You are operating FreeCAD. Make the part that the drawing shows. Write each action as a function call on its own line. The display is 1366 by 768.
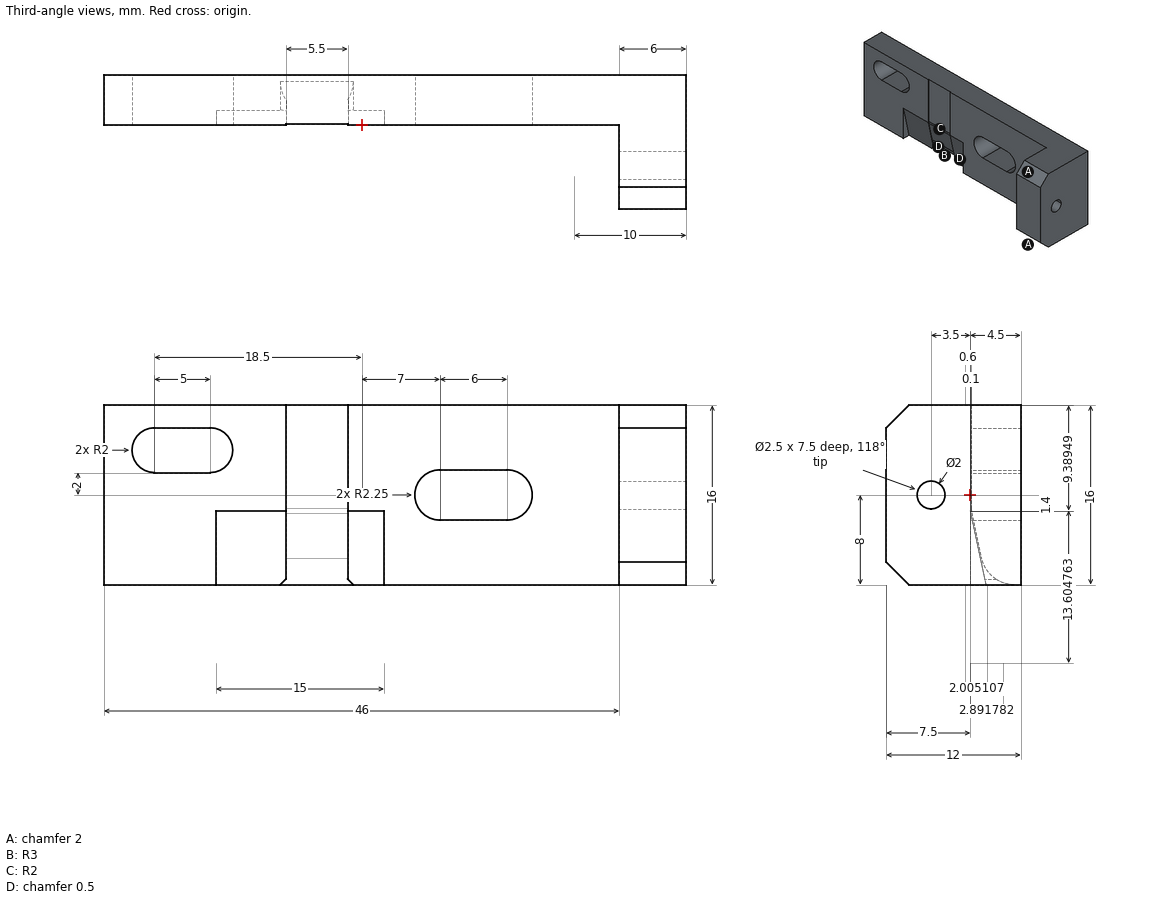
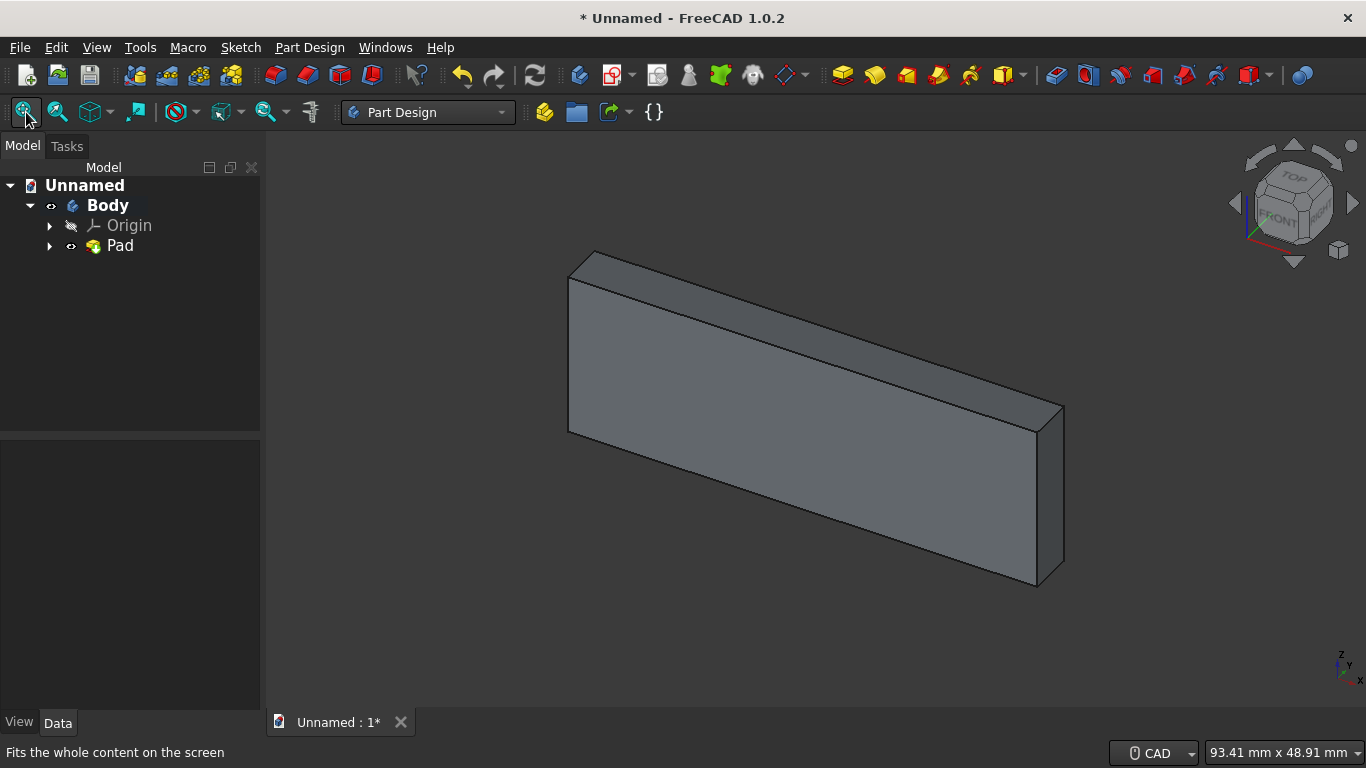
click(1051, 474)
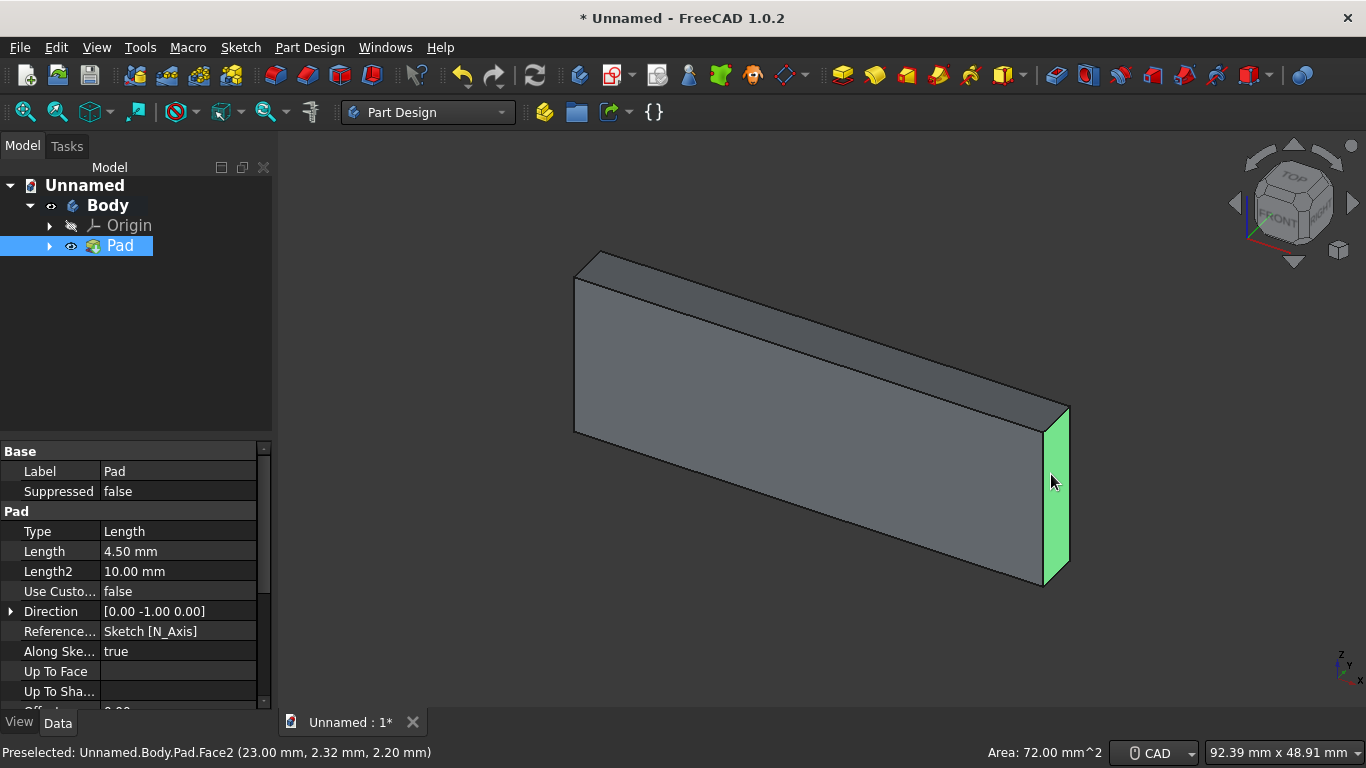
click(612, 76)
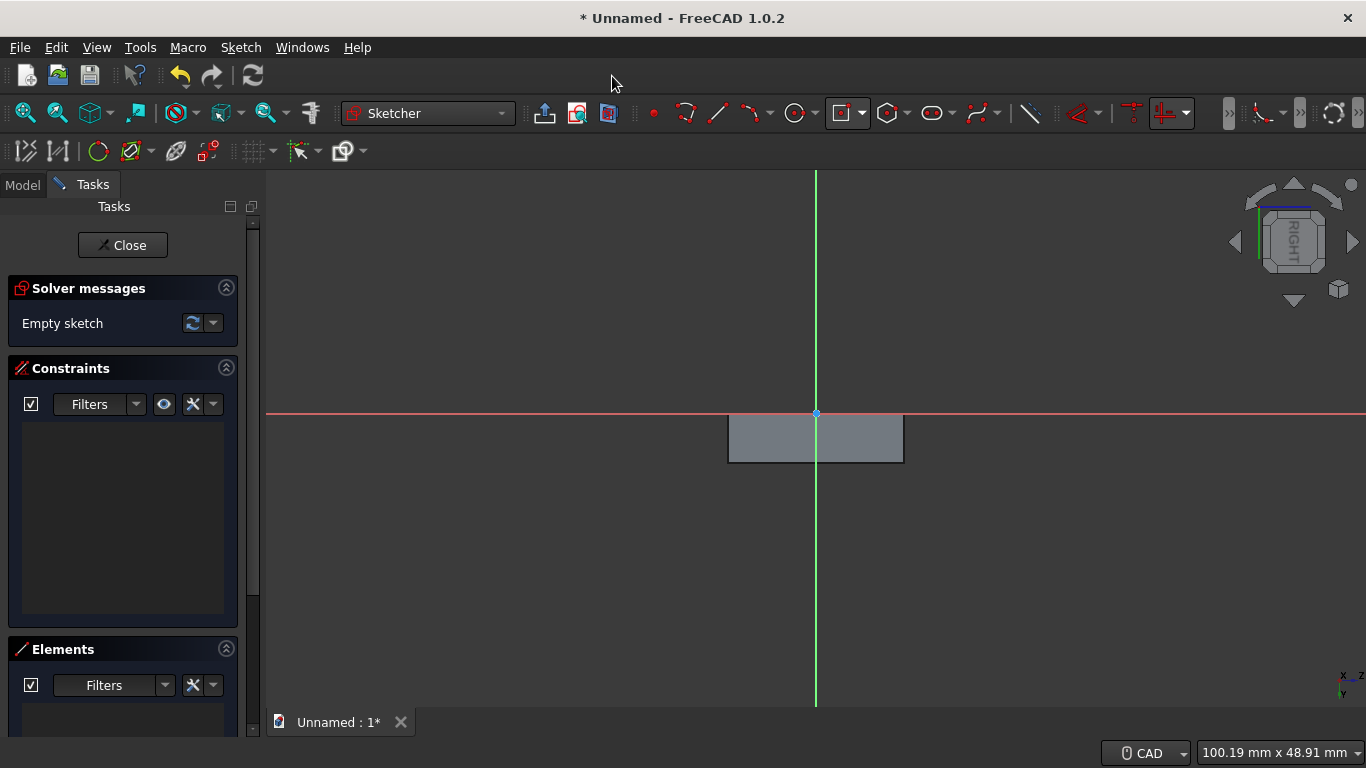
scroll(856, 373, up, 5)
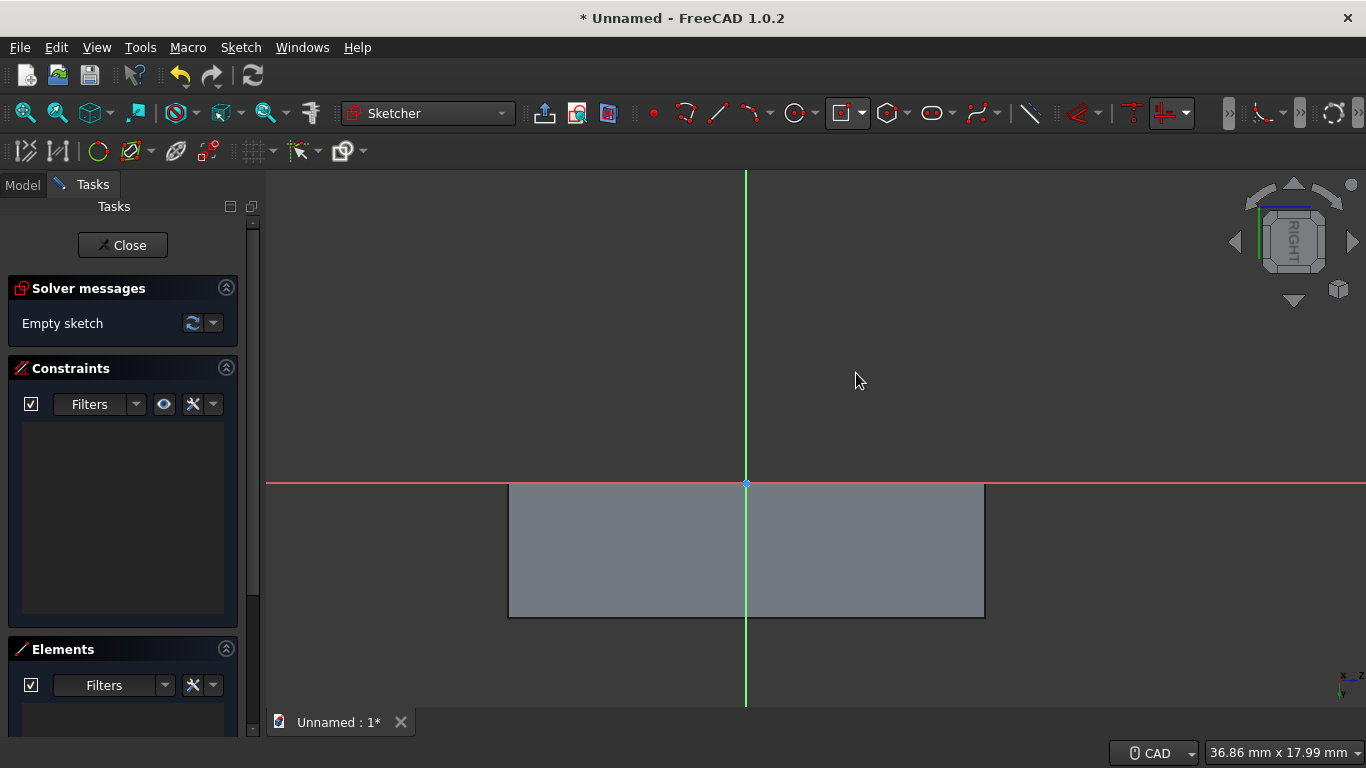
key(g)
key(r)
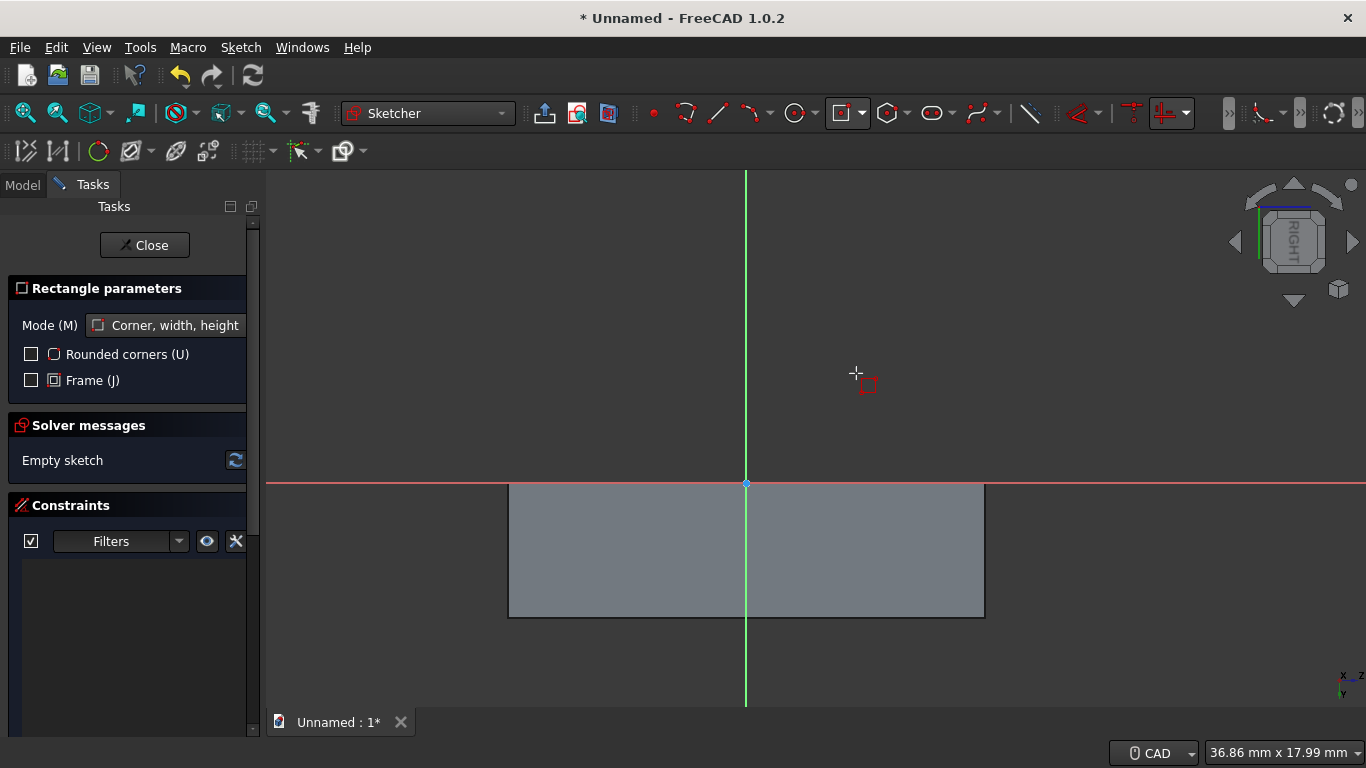
click(508, 259)
click(985, 618)
key(Escape)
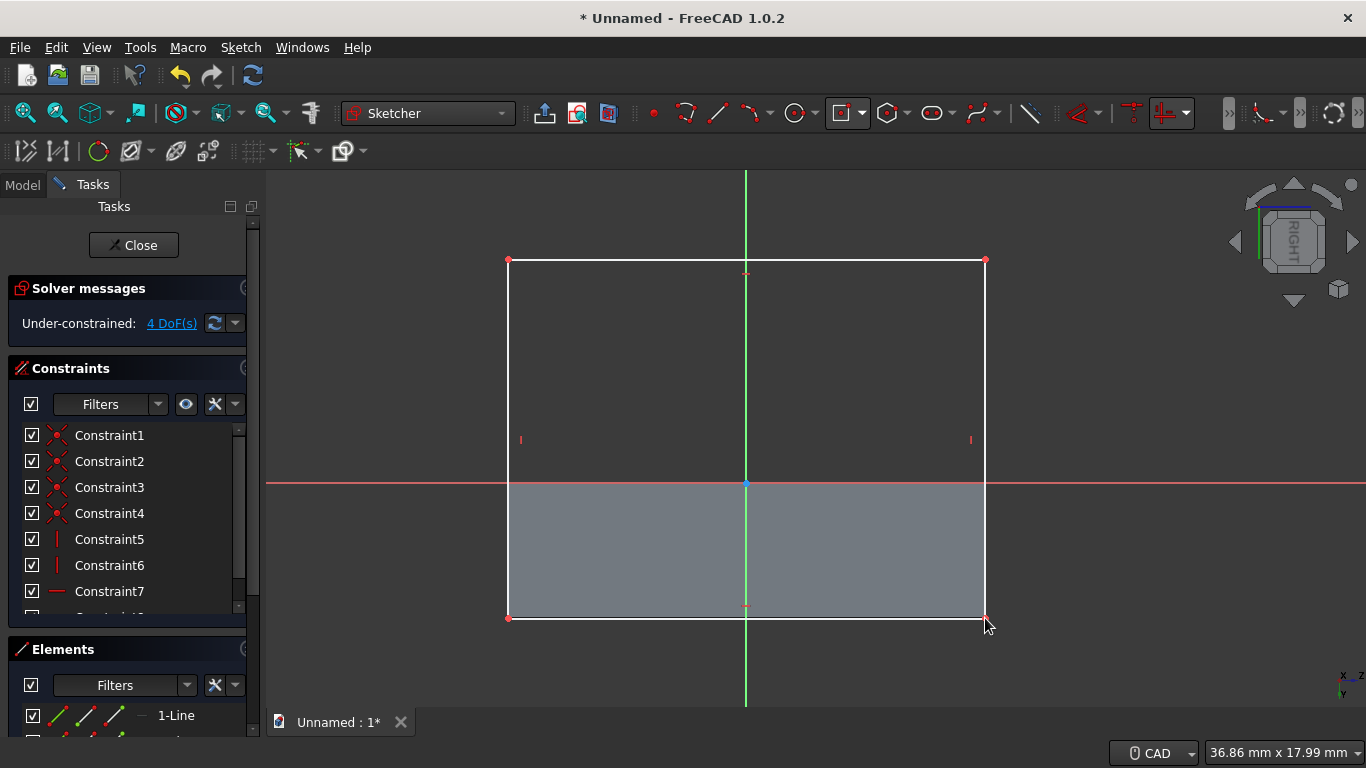
click(1078, 114)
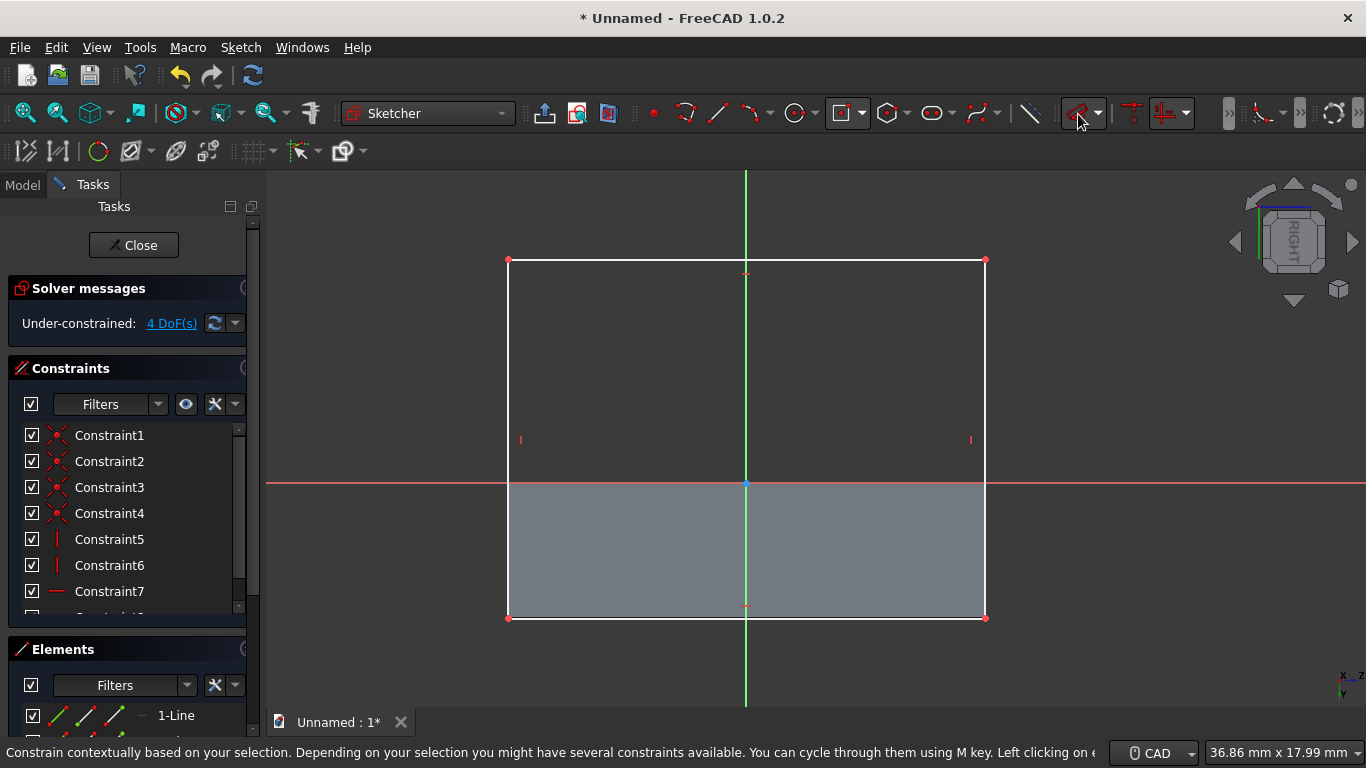
click(508, 368)
click(474, 439)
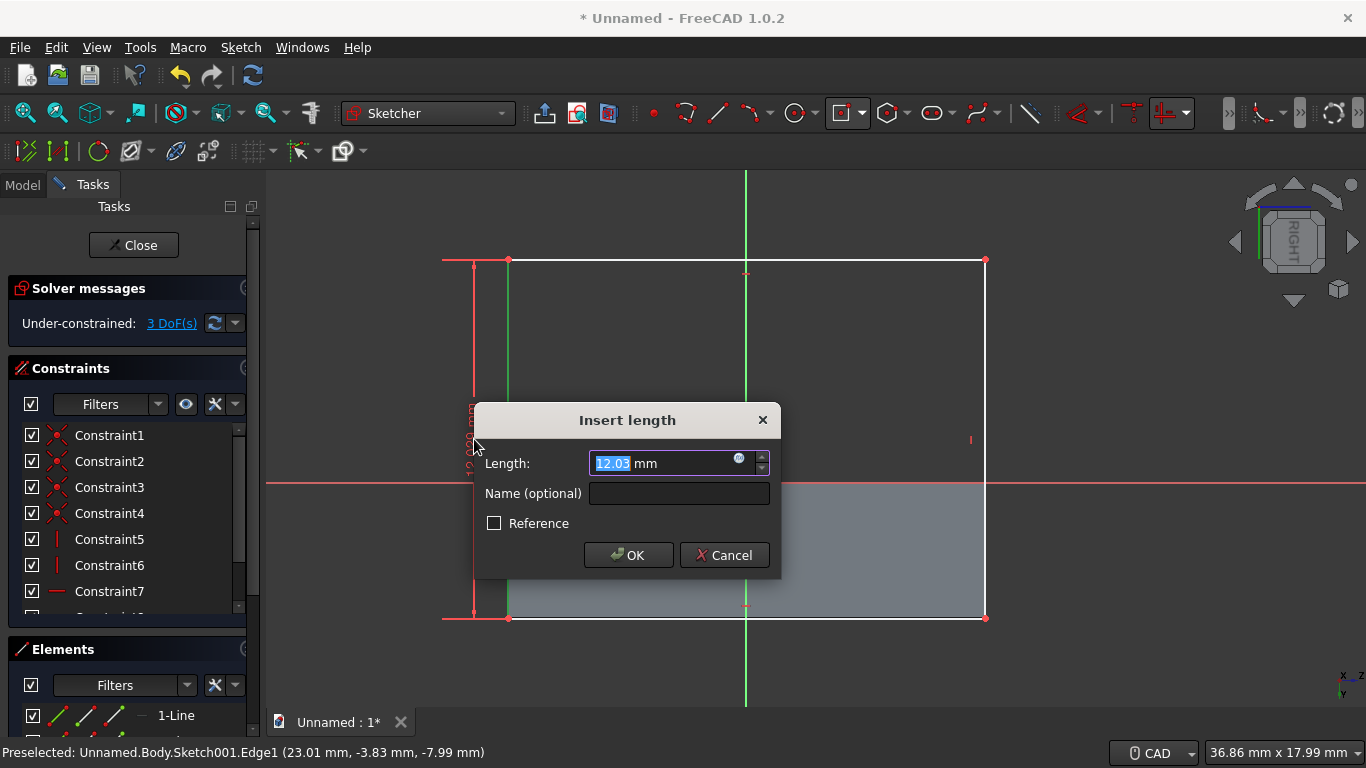
text(12)
key(Return)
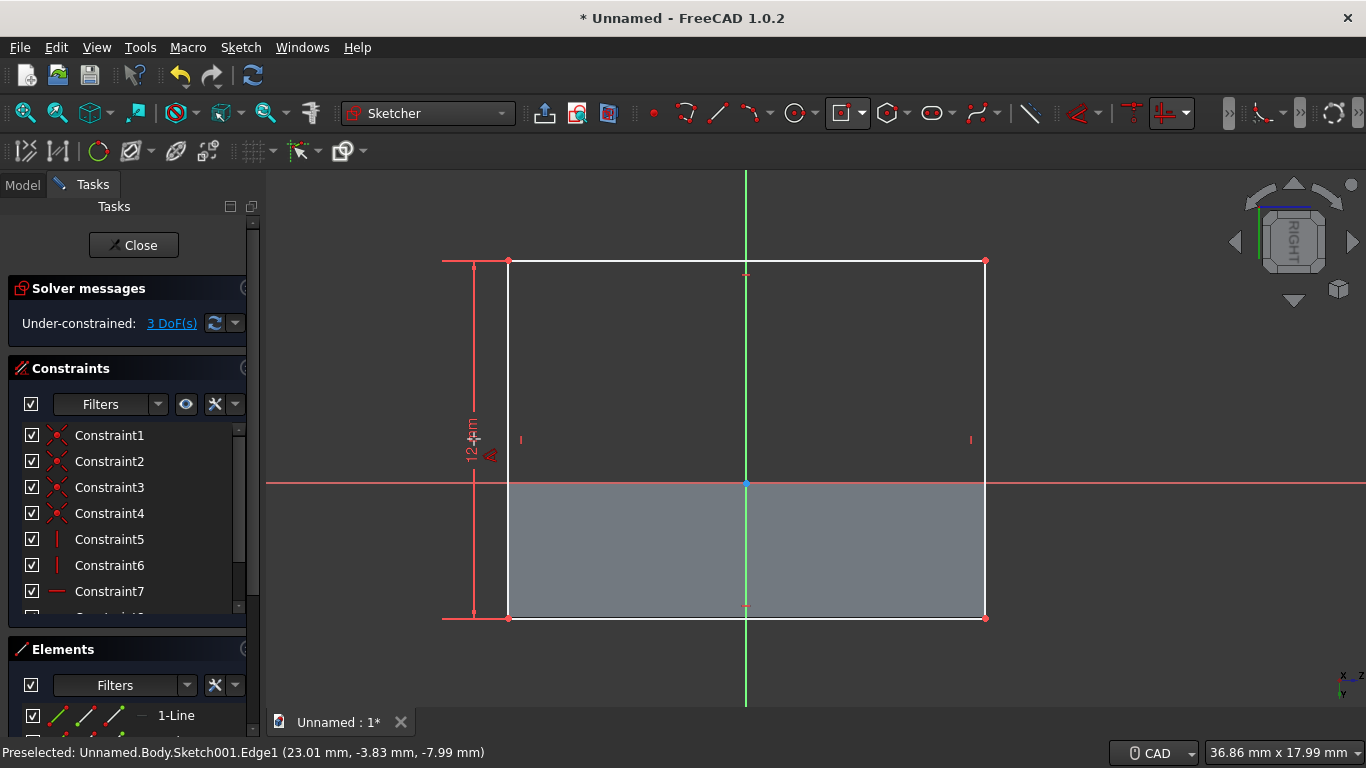
click(651, 619)
click(637, 653)